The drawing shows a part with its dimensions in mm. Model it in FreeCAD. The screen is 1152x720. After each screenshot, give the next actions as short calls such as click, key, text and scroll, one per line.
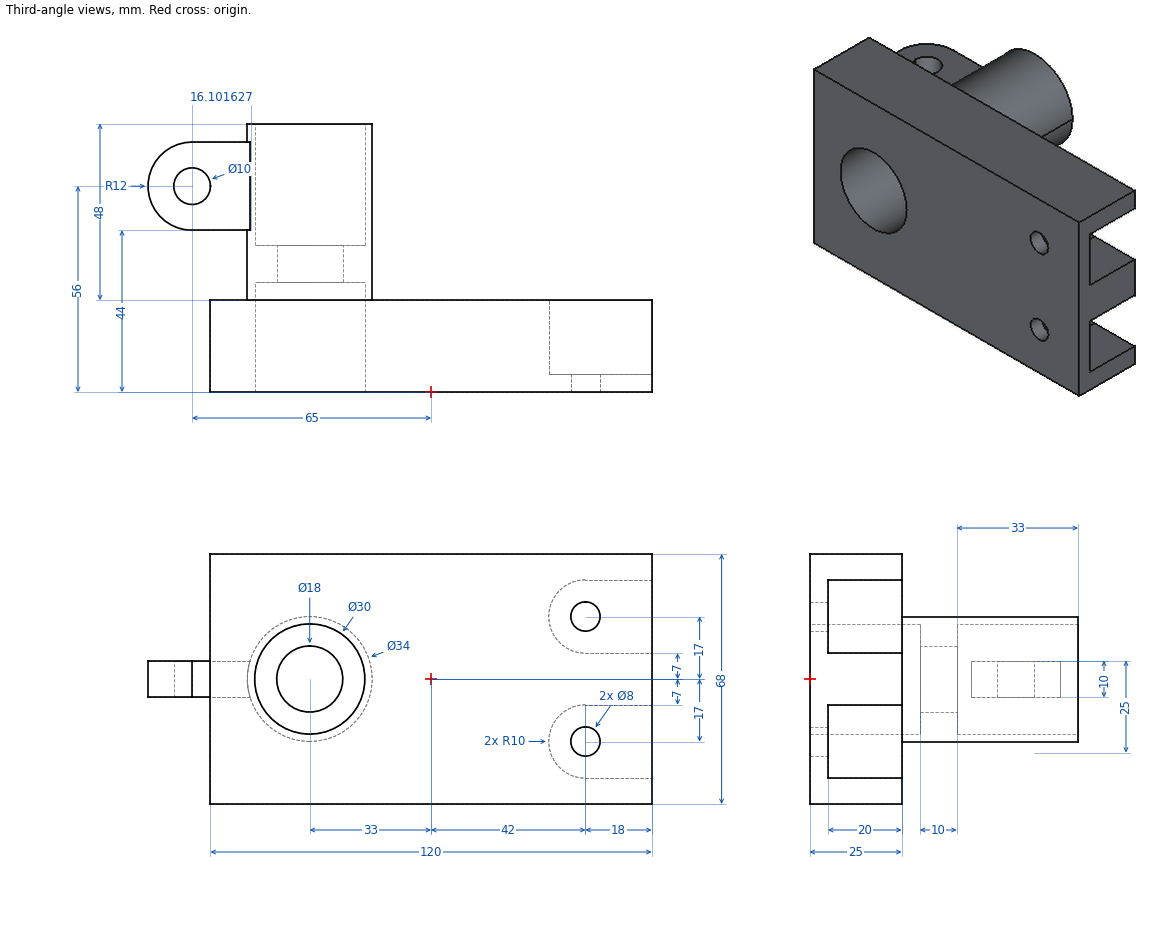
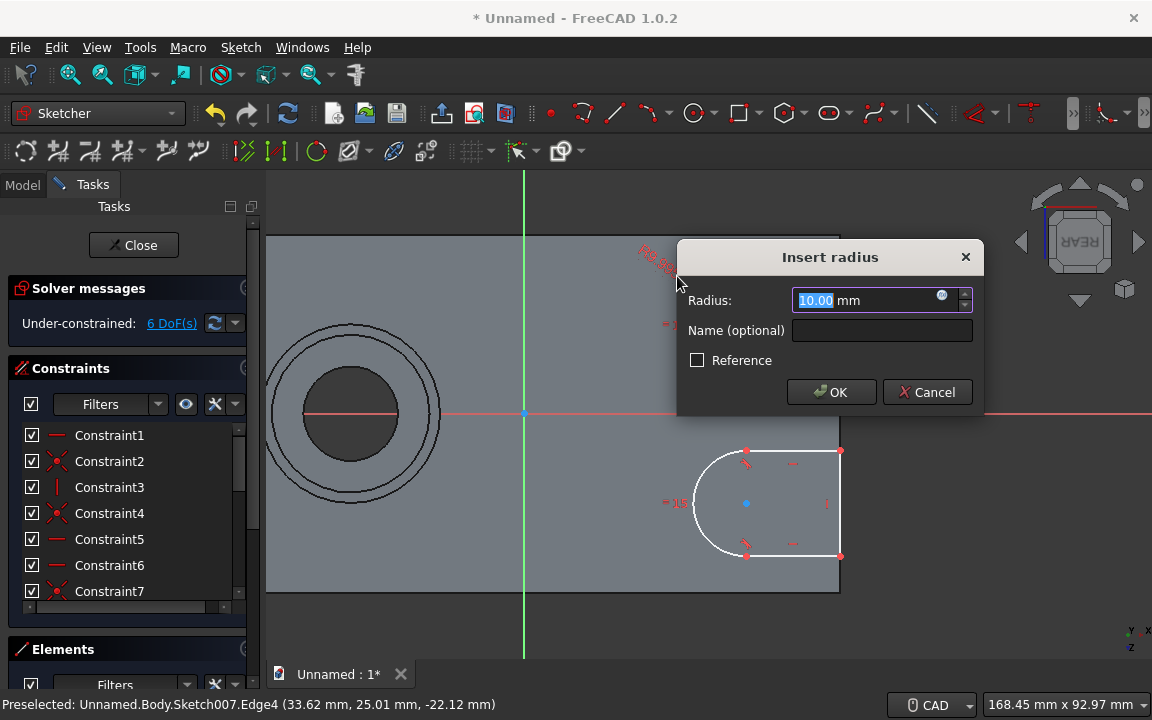
text(10)
key(Return)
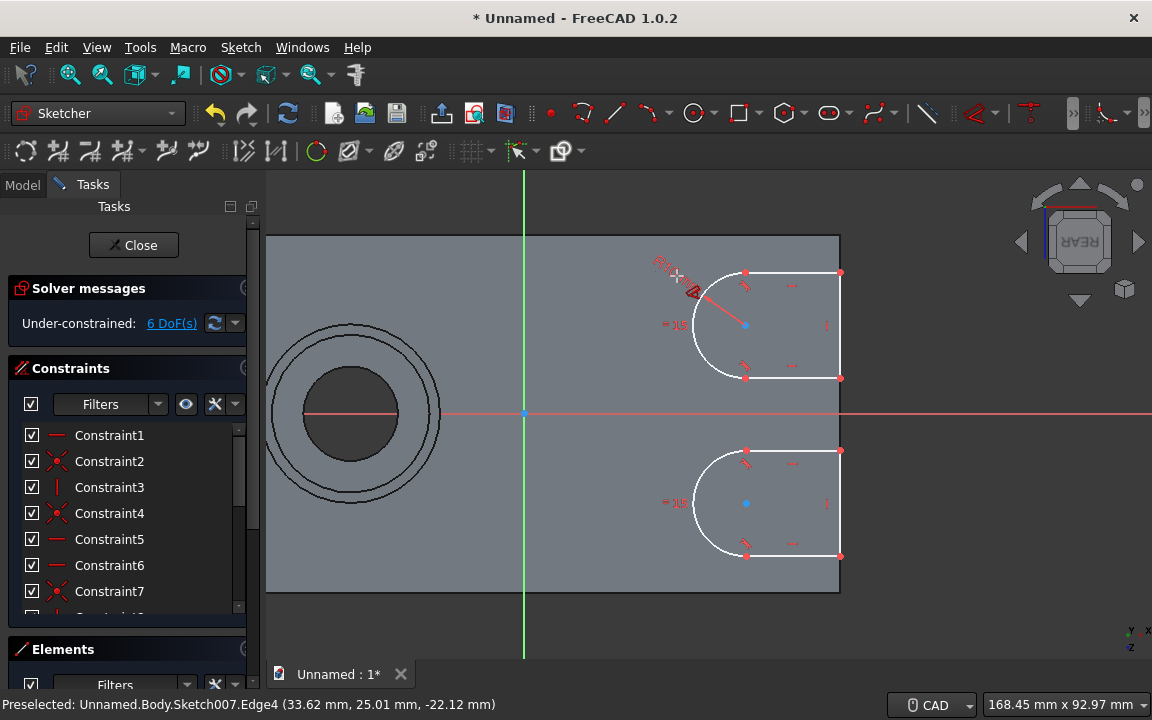
click(774, 378)
click(793, 344)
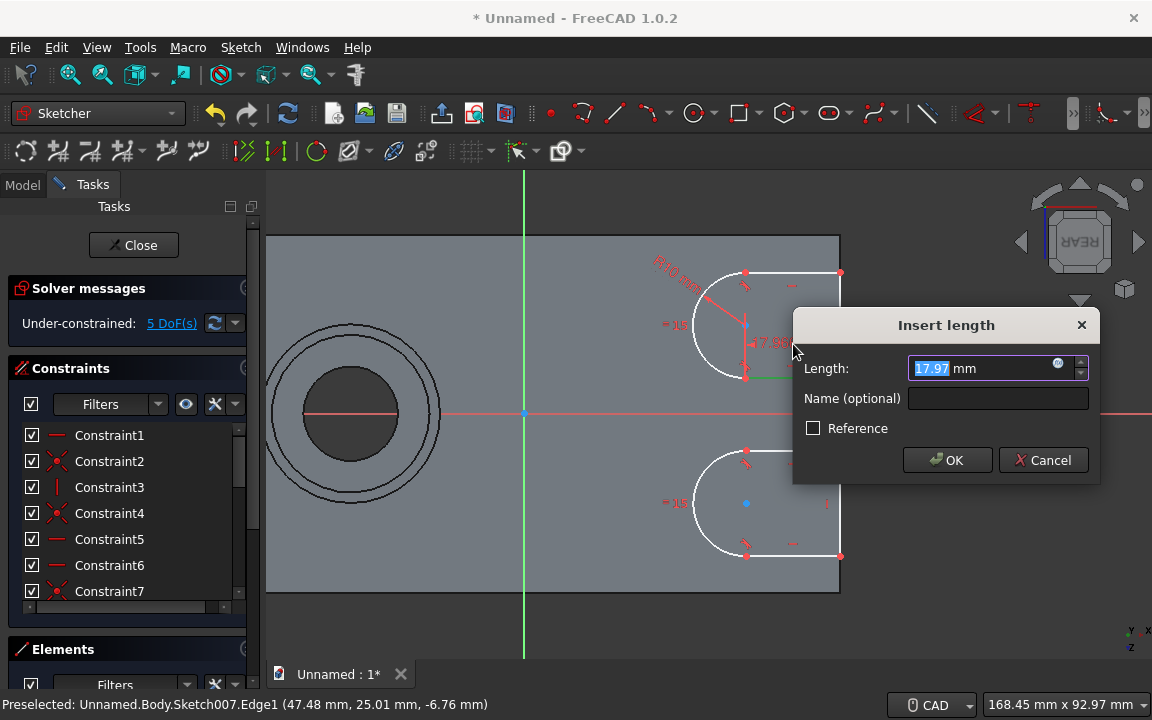
text(18)
key(Return)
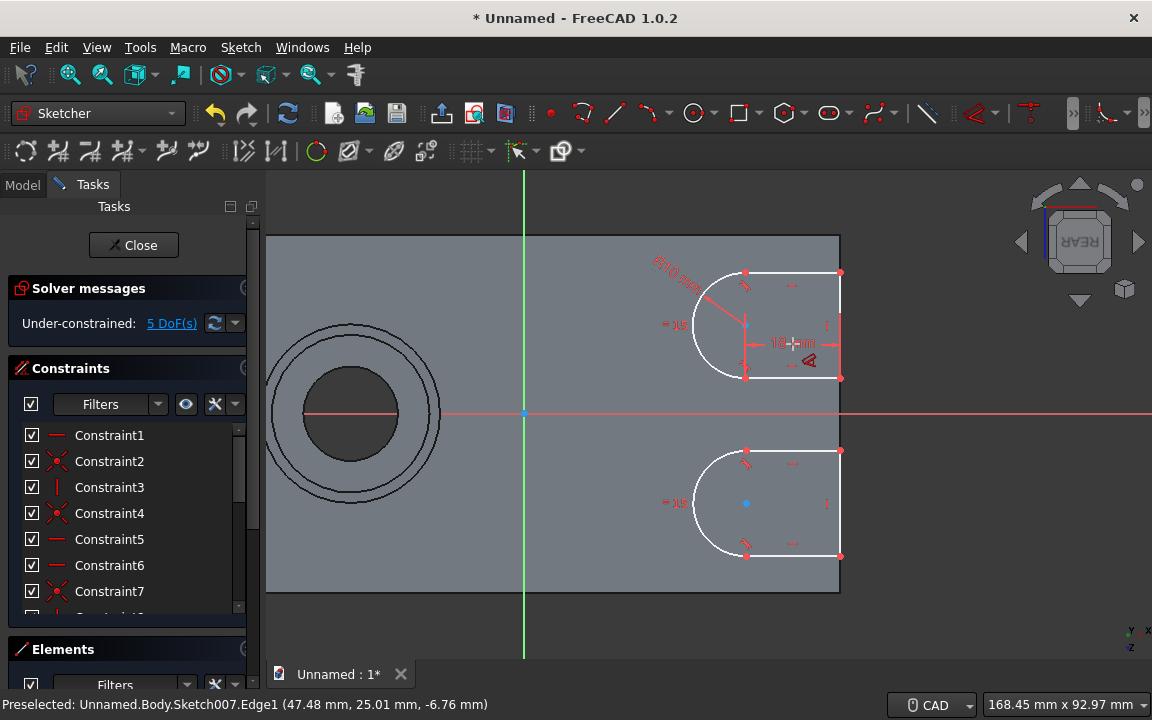
click(774, 556)
click(793, 590)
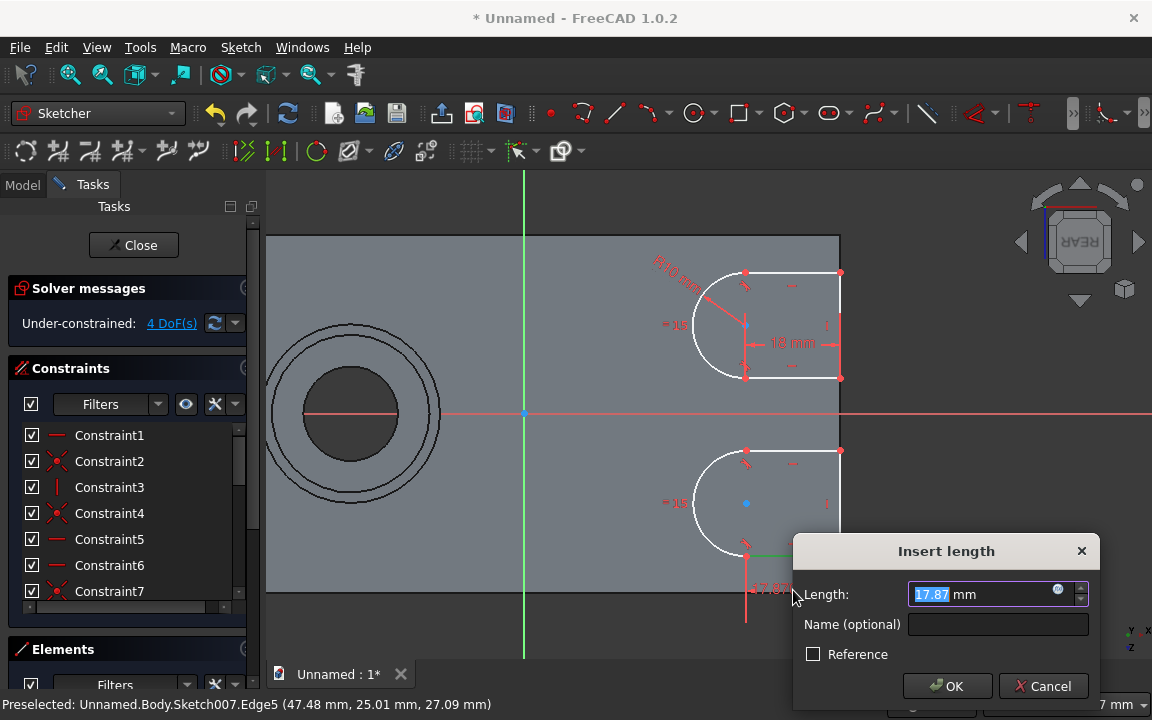
text(18)
key(Return)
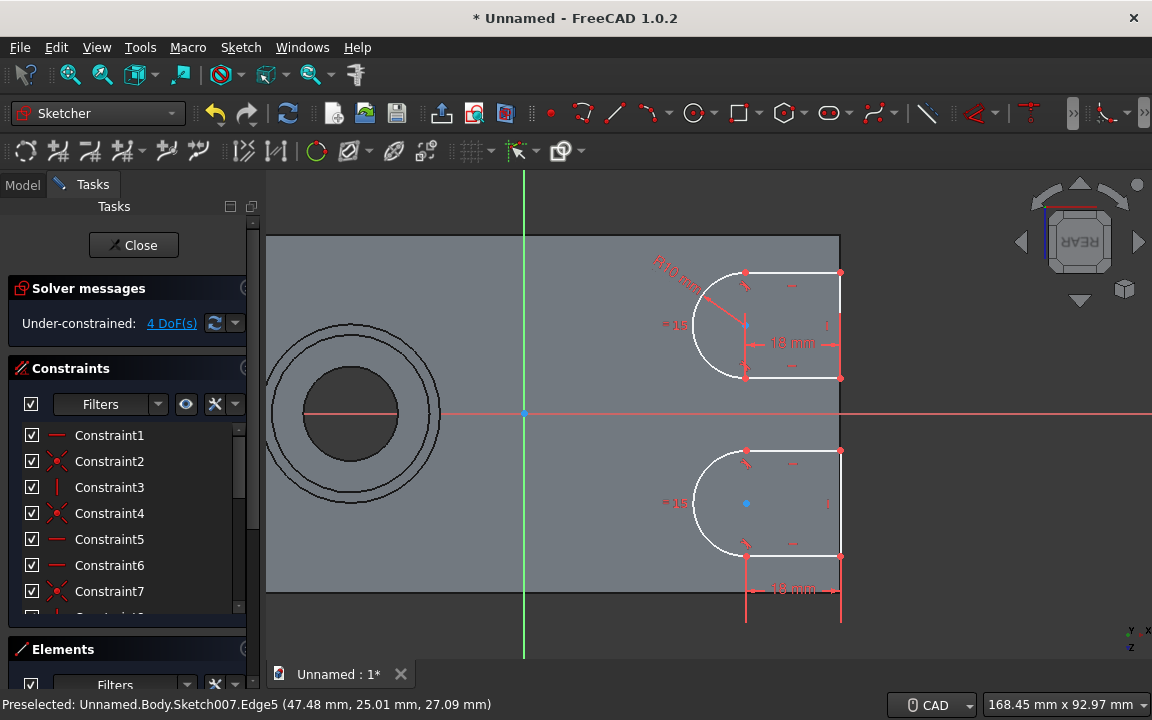
click(745, 378)
click(490, 396)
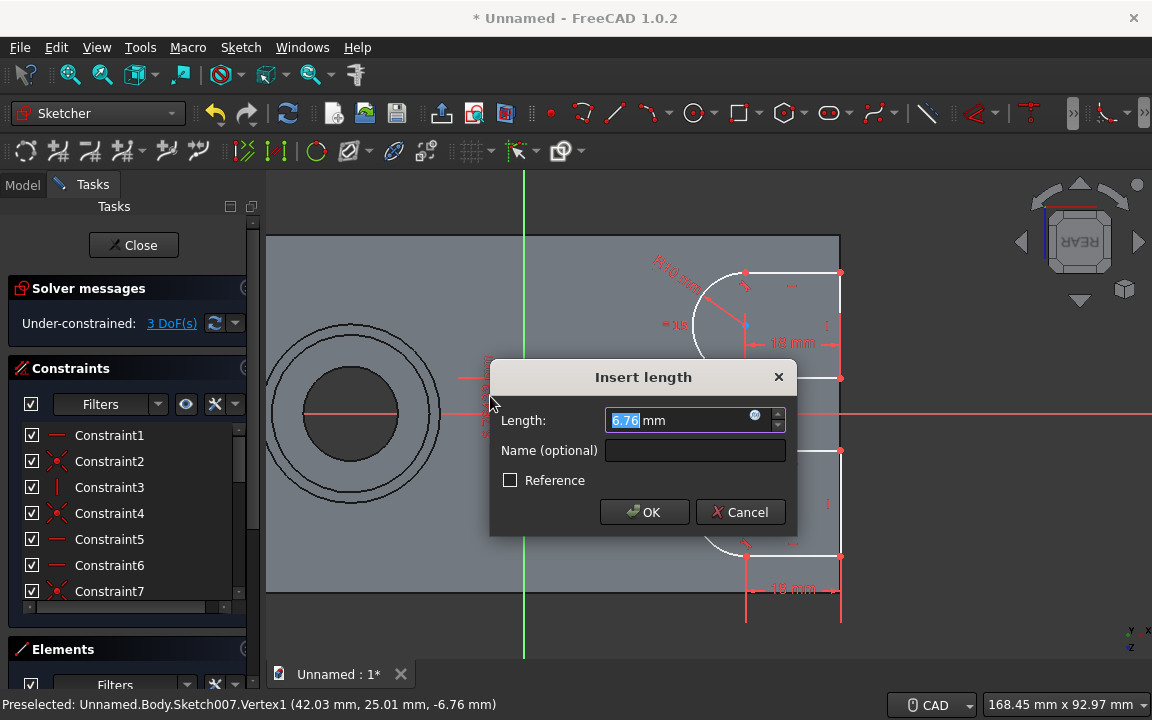
text(7)
key(Return)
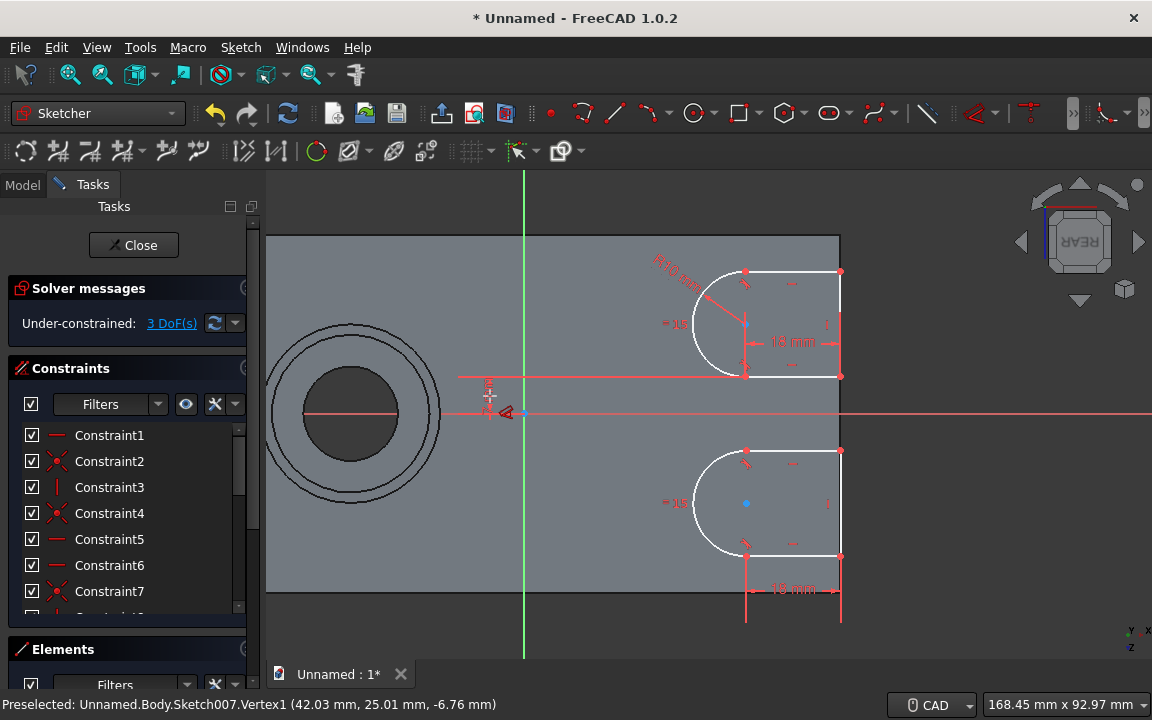
click(841, 451)
click(875, 432)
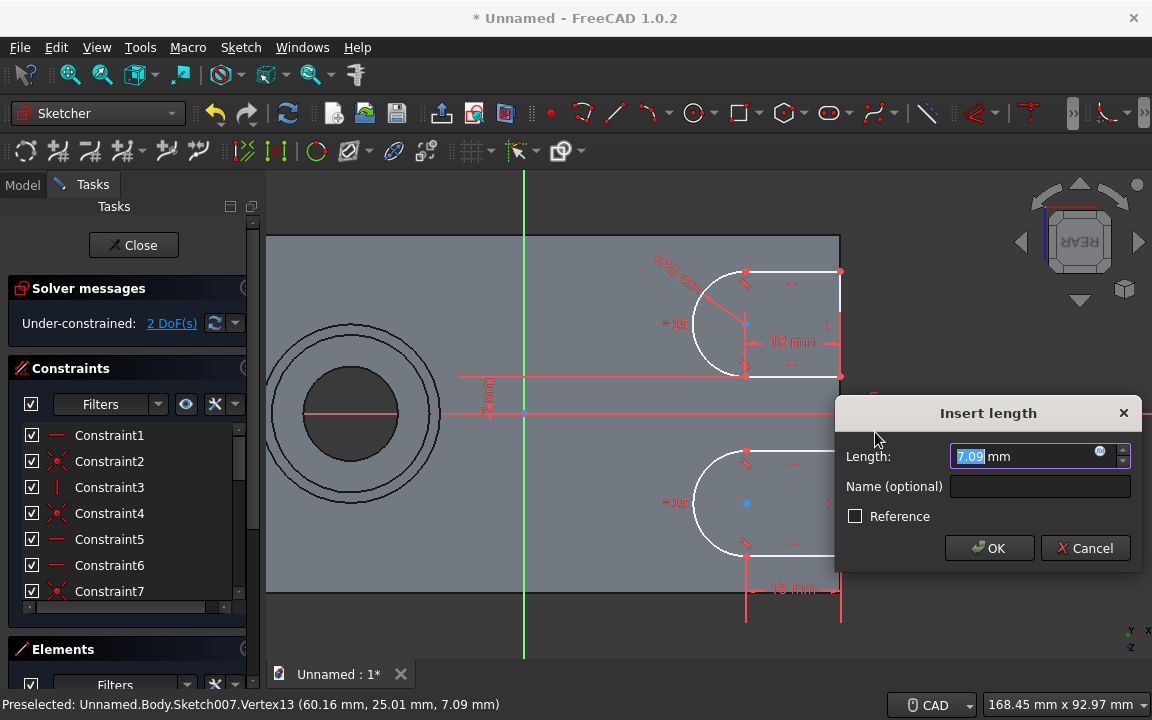
text(7)
key(Return)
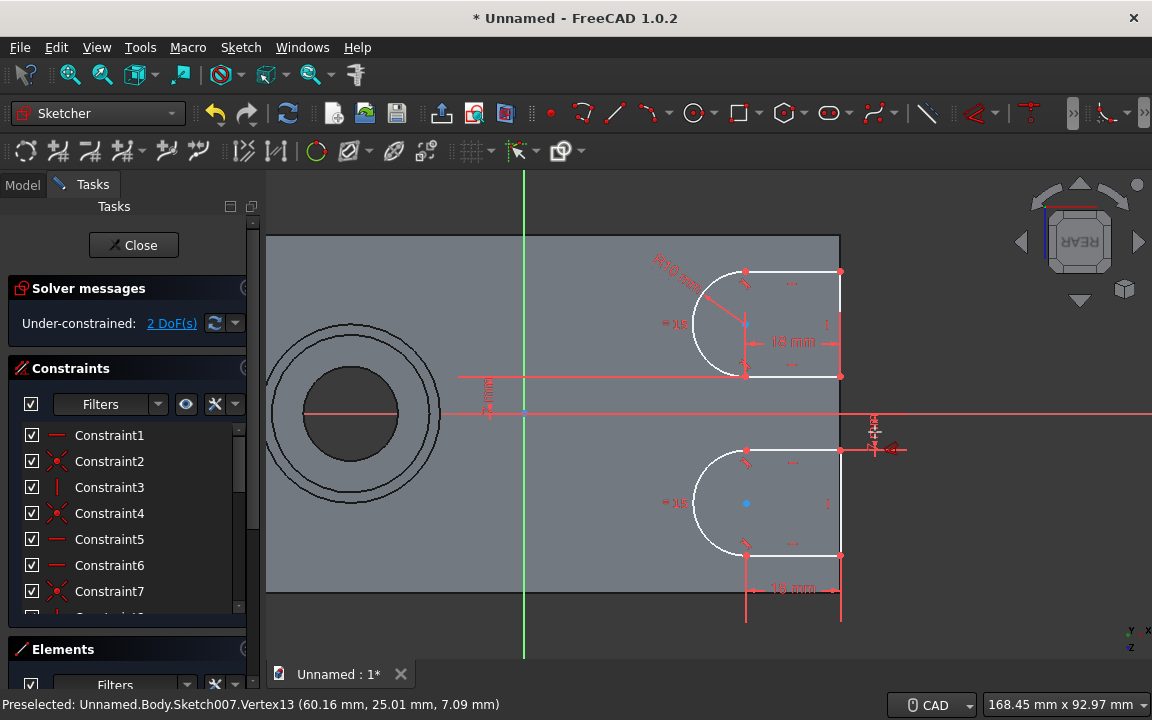
click(745, 377)
click(635, 343)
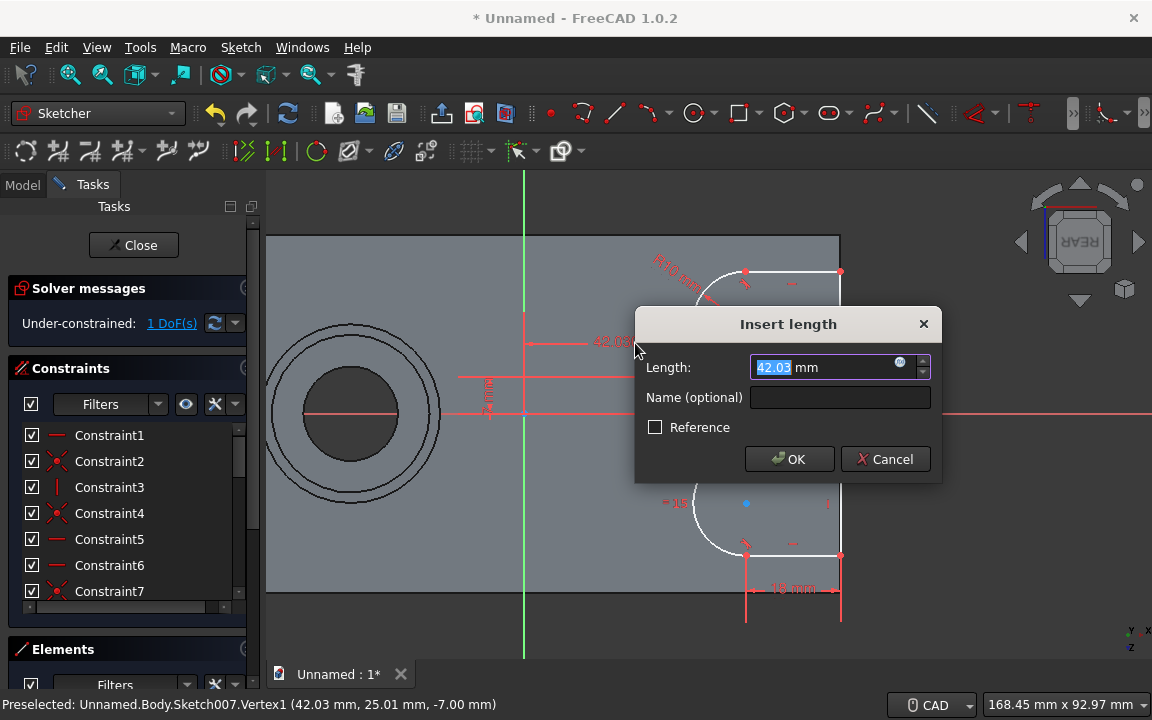
text(42)
key(Return)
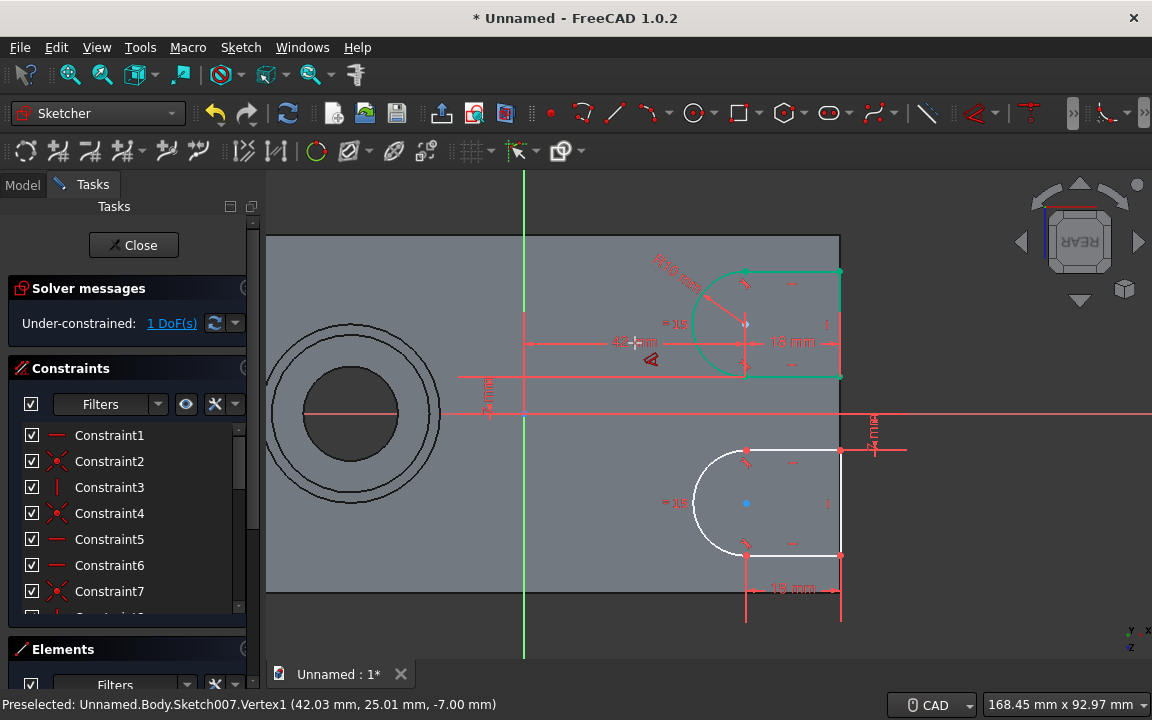
click(746, 556)
click(635, 590)